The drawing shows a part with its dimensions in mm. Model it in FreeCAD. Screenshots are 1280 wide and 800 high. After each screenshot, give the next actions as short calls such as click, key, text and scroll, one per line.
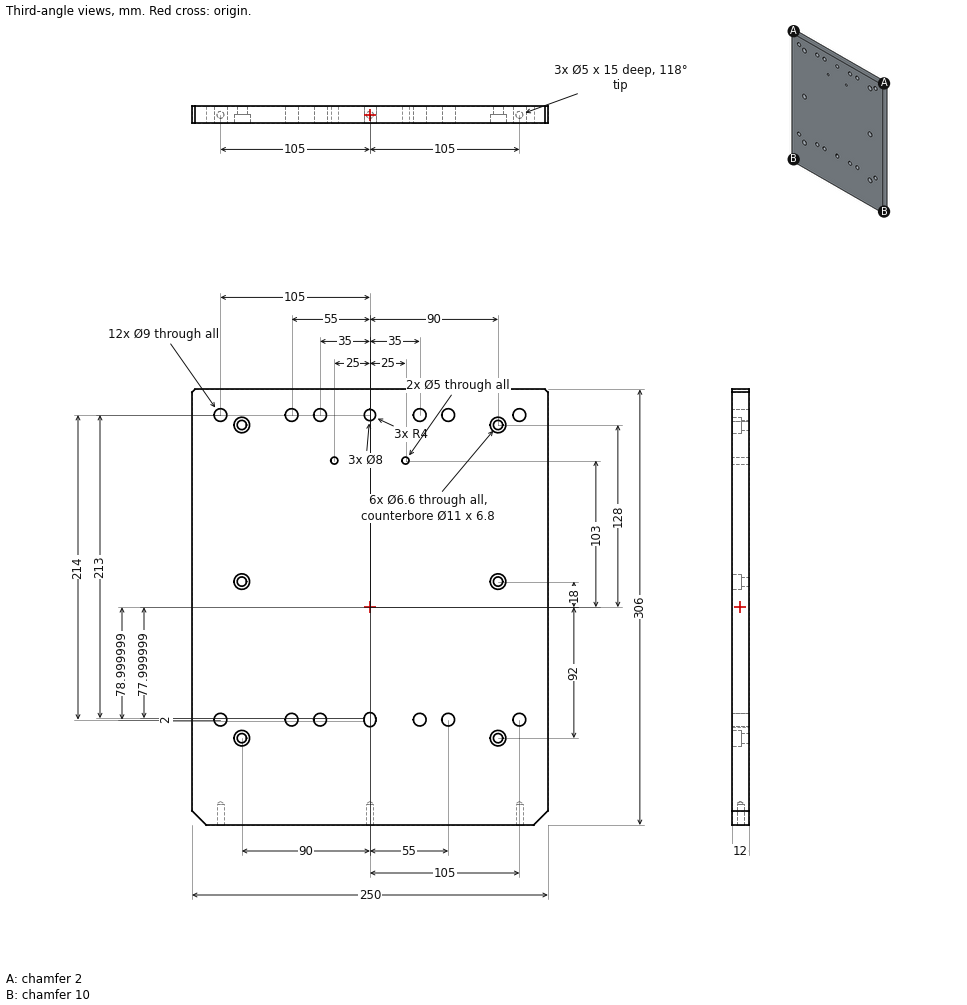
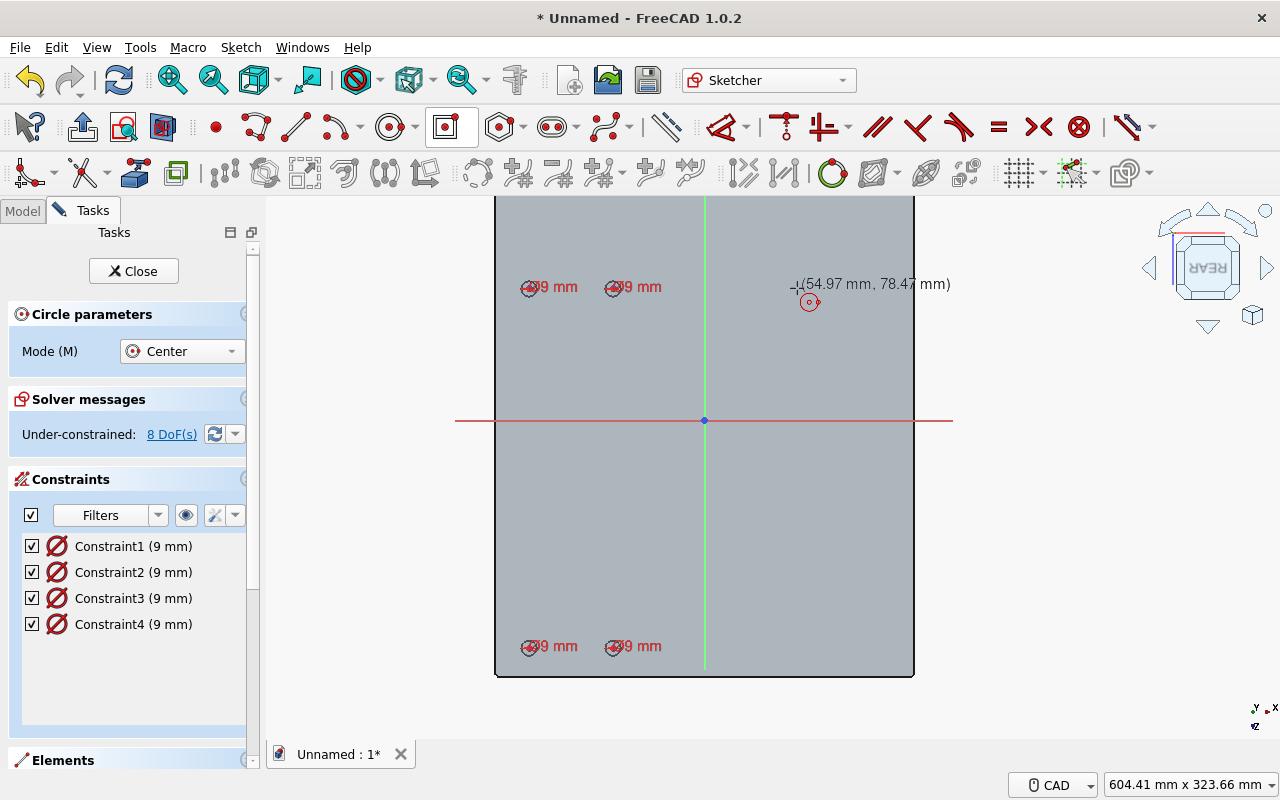
click(797, 288)
move(802, 283)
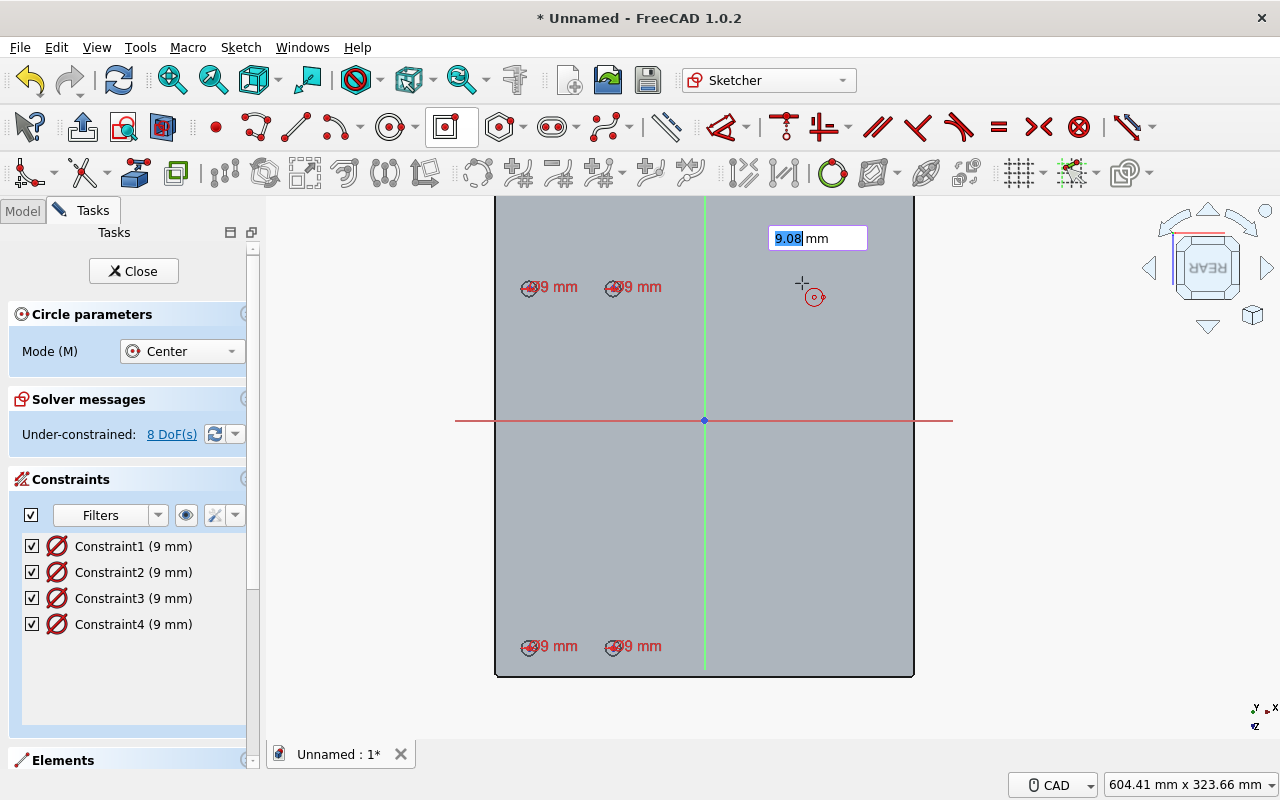
text(9)
key(Return)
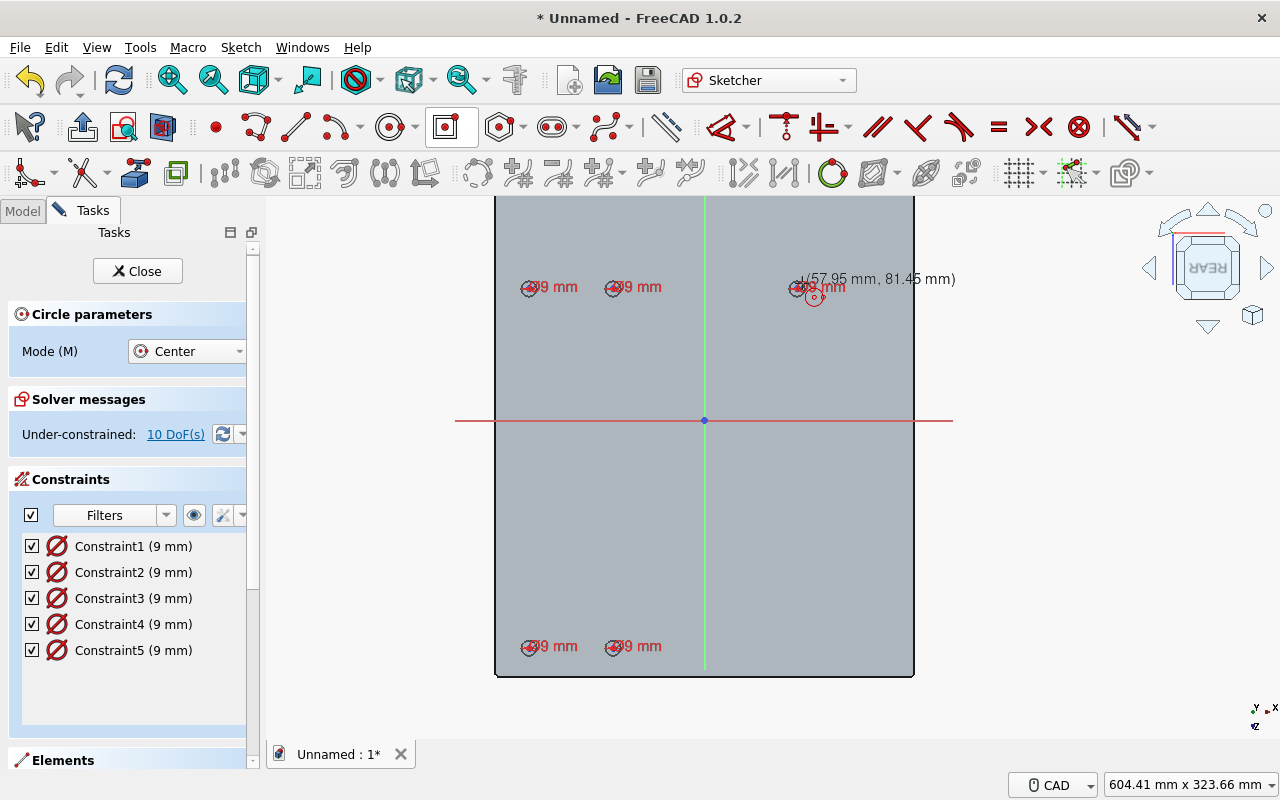
scroll(881, 288, up, 6)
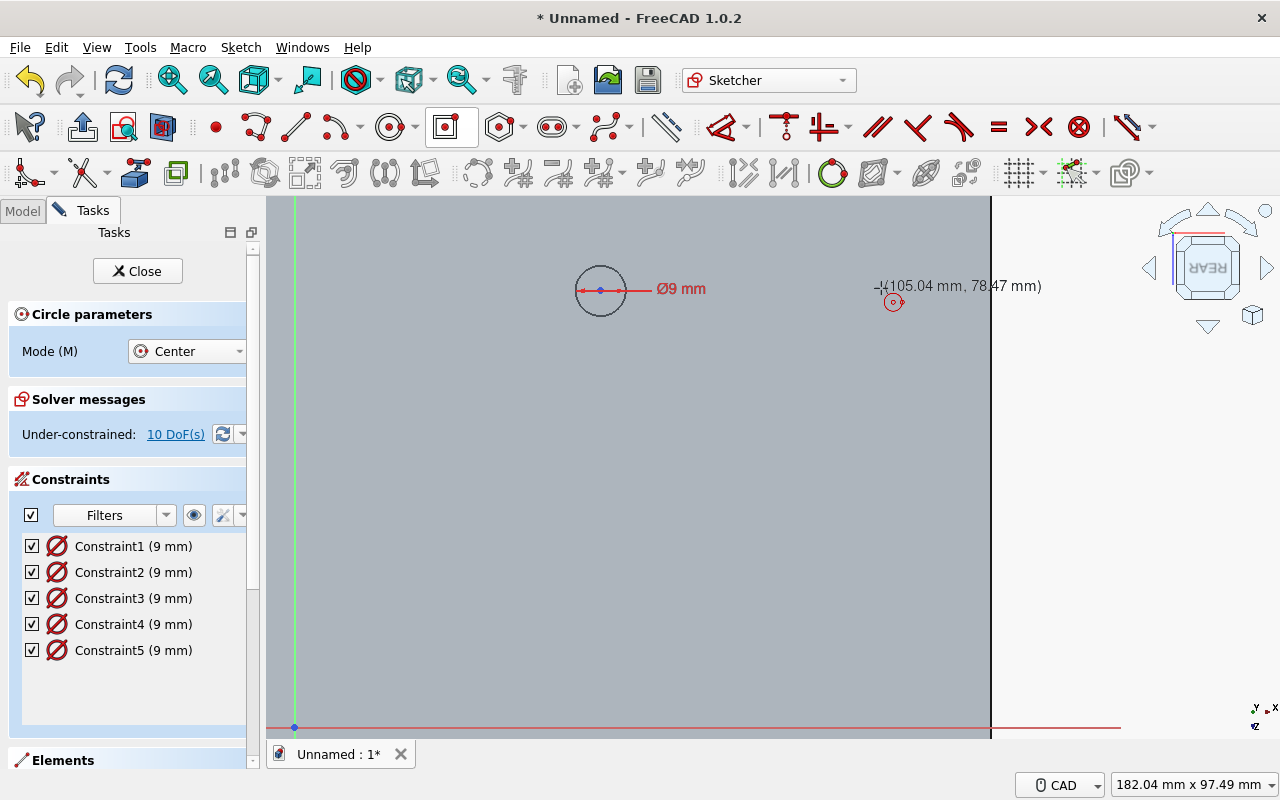
scroll(881, 288, down, 6)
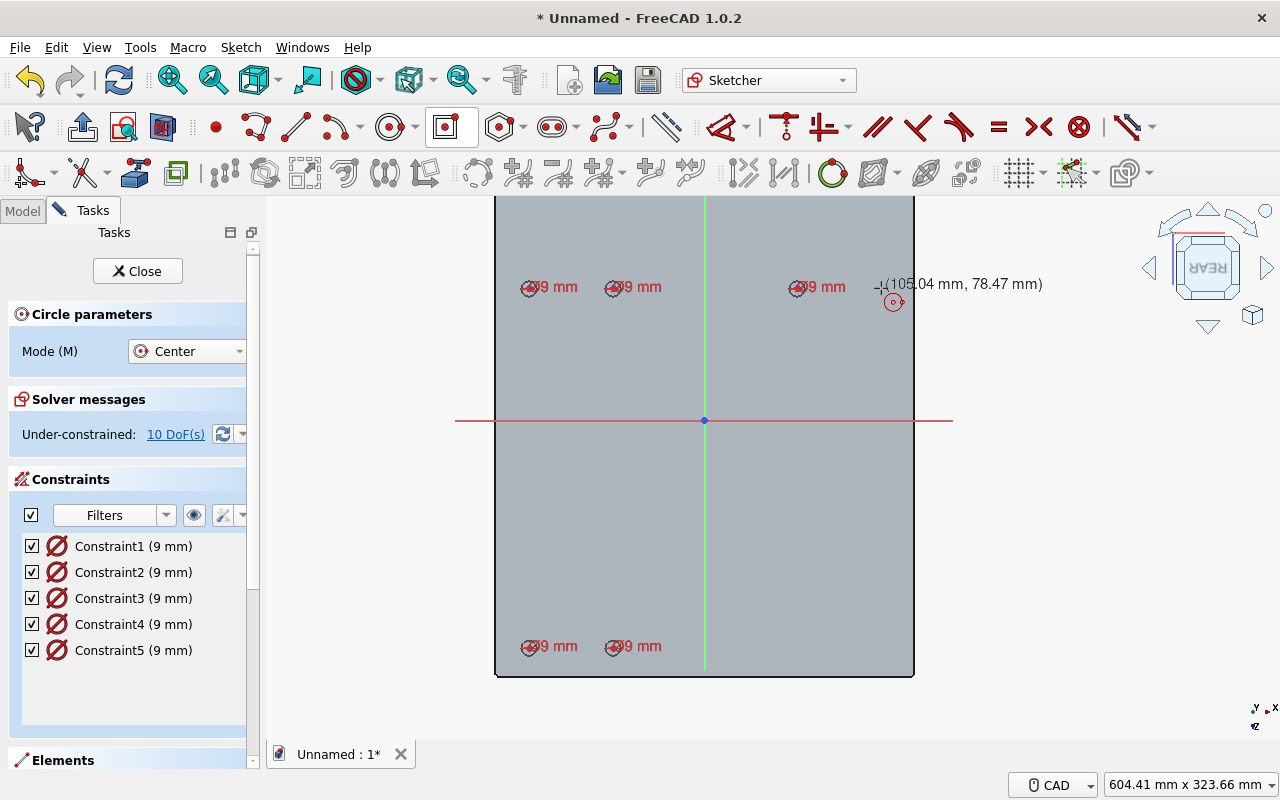
click(881, 288)
move(886, 283)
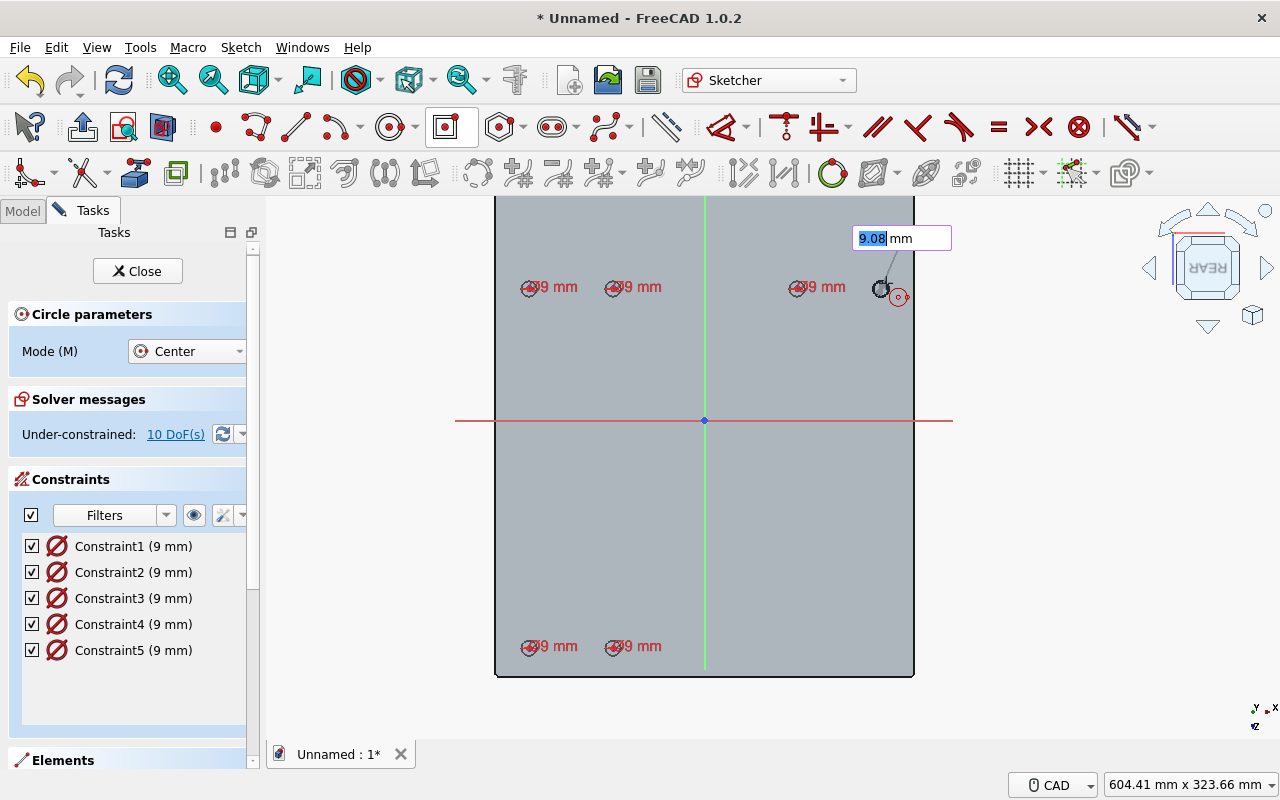
text(9)
key(Return)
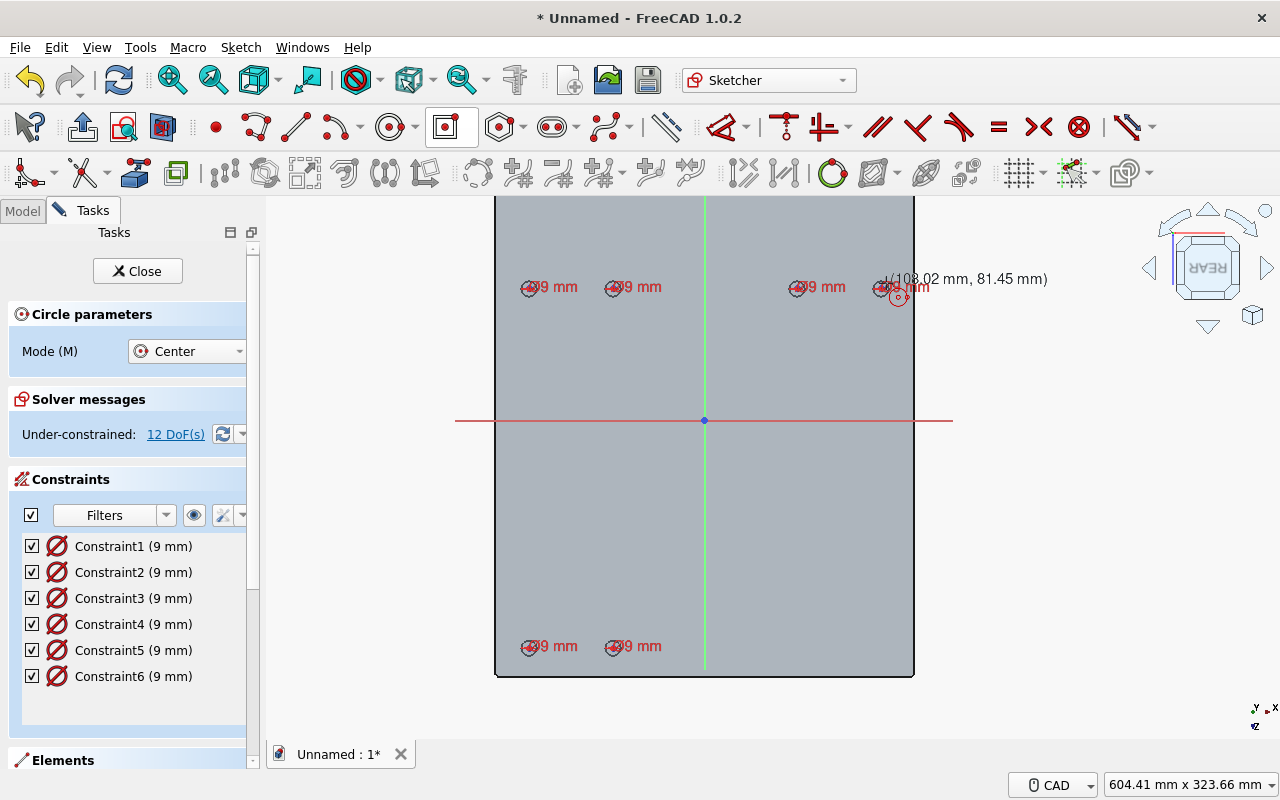
scroll(797, 647, up, 6)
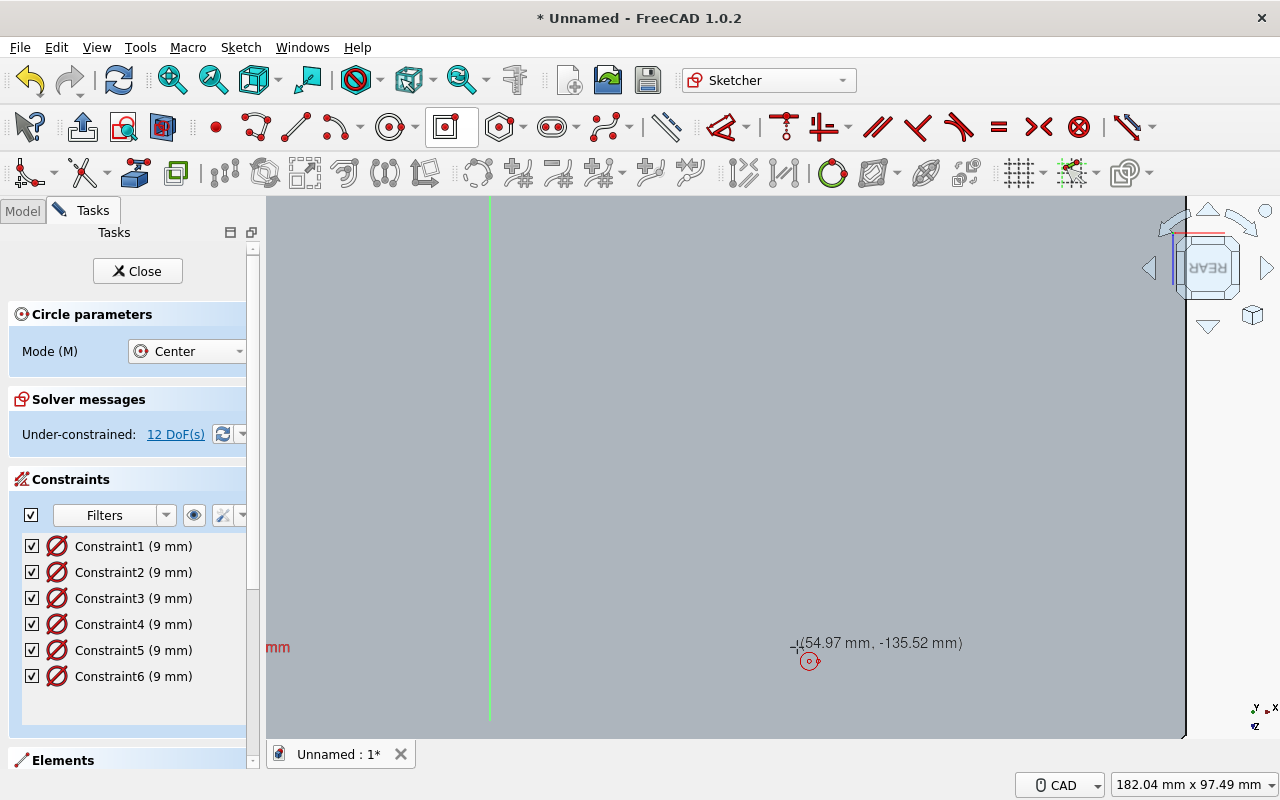
scroll(797, 648, down, 6)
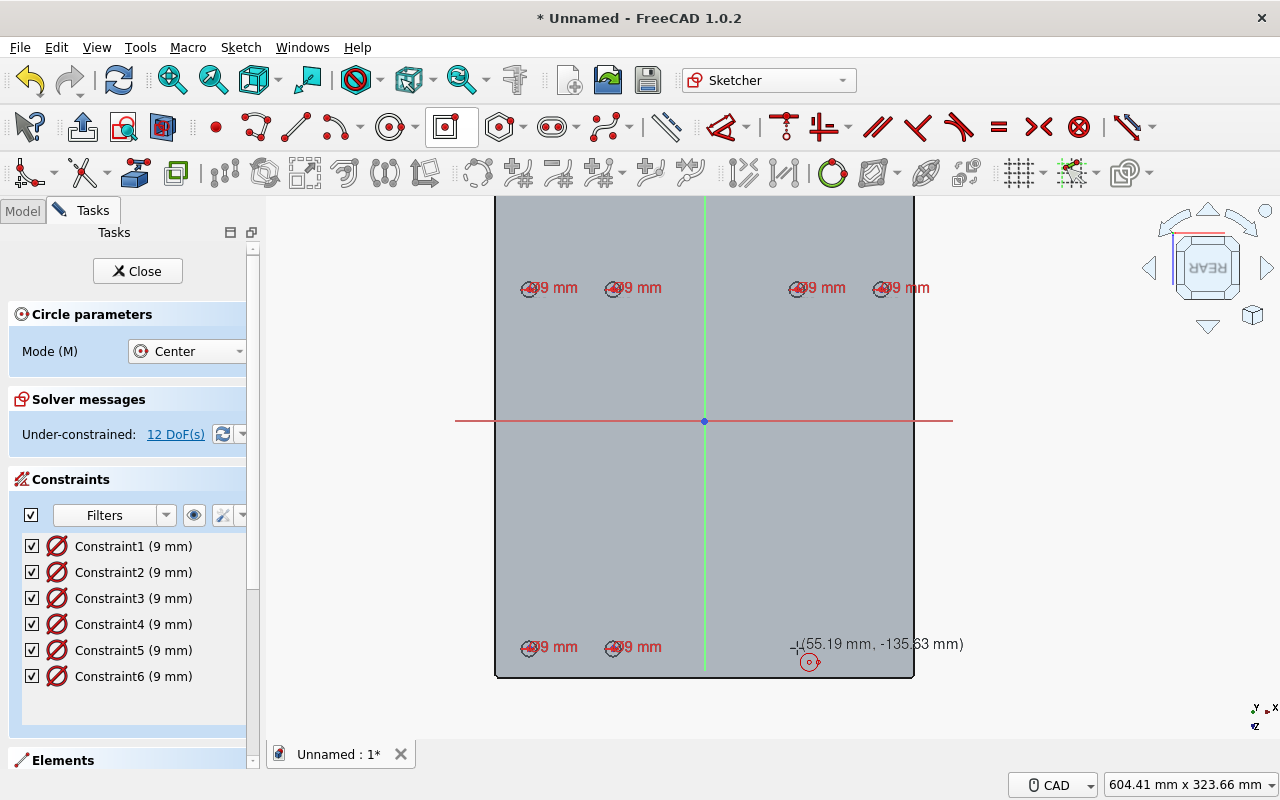
click(797, 648)
move(802, 642)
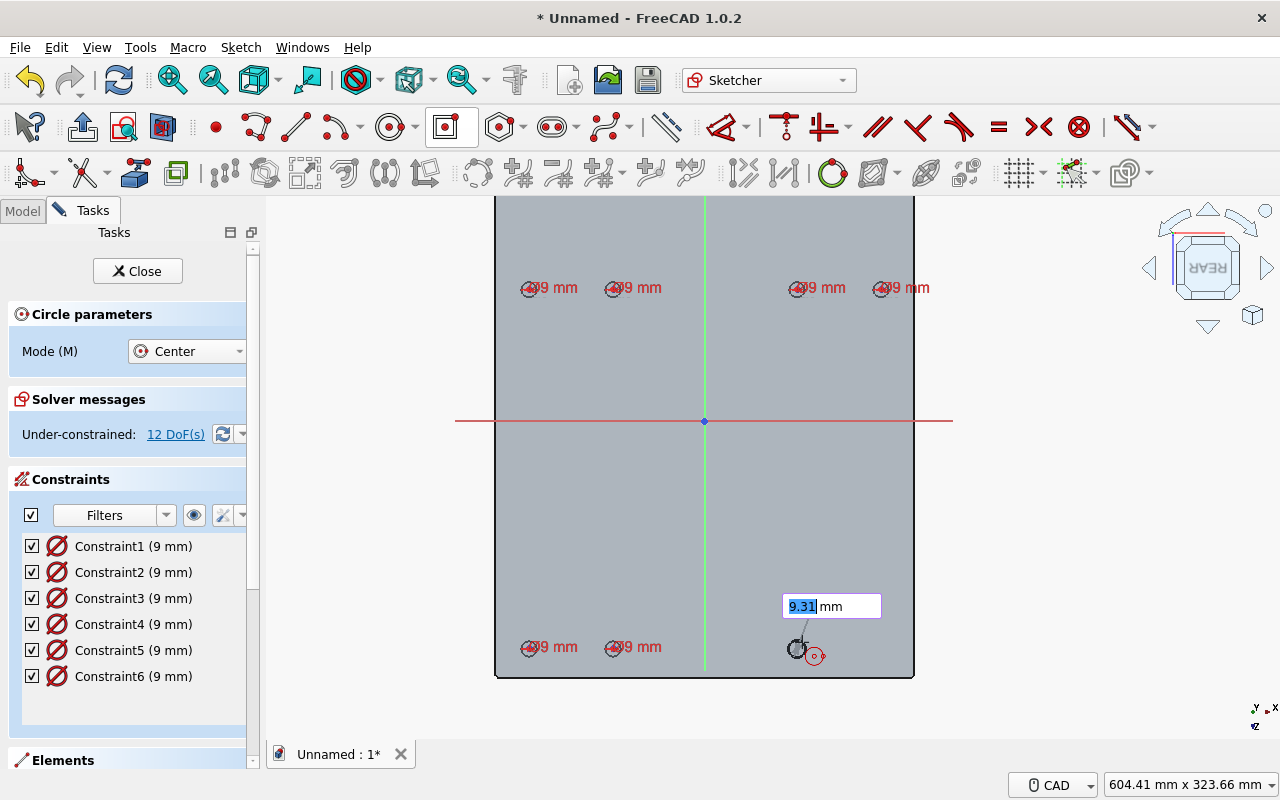
text(9)
key(Return)